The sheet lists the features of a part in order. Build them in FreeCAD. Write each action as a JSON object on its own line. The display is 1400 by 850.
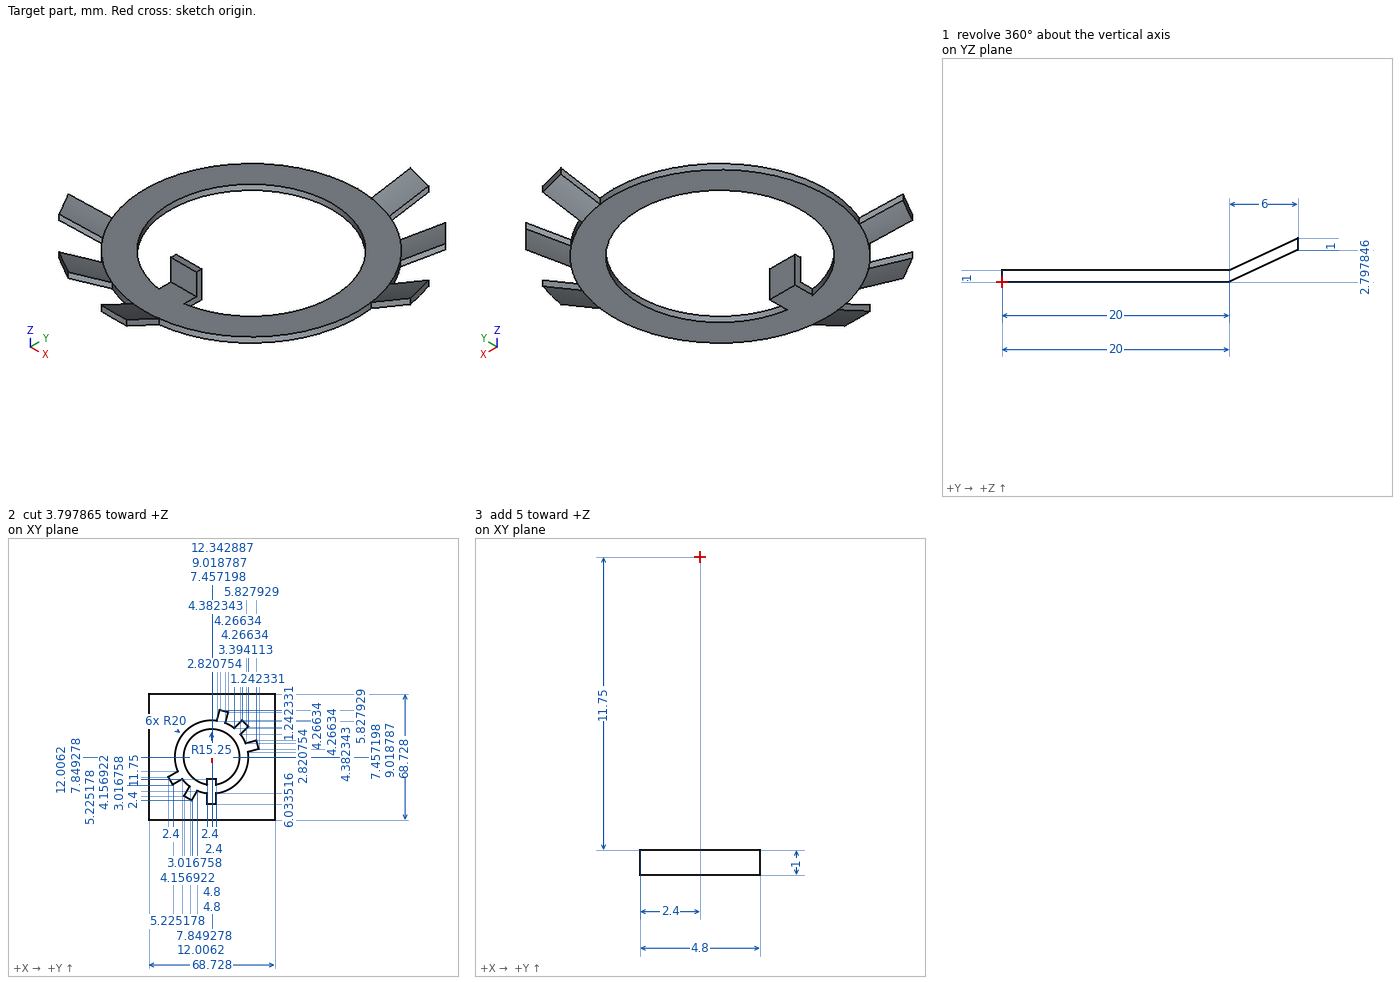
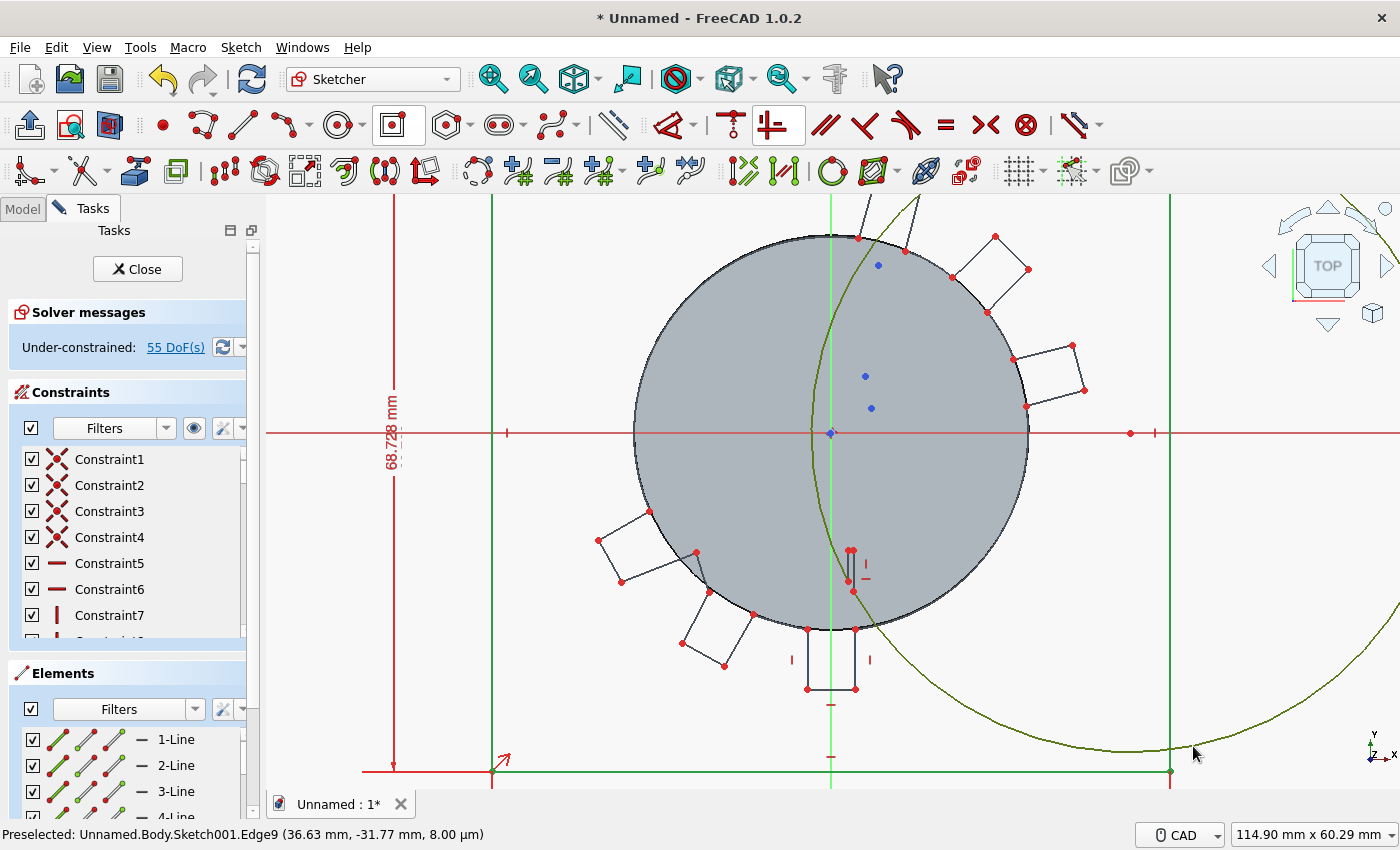
{"action": "left_click", "coordinate": [738, 260]}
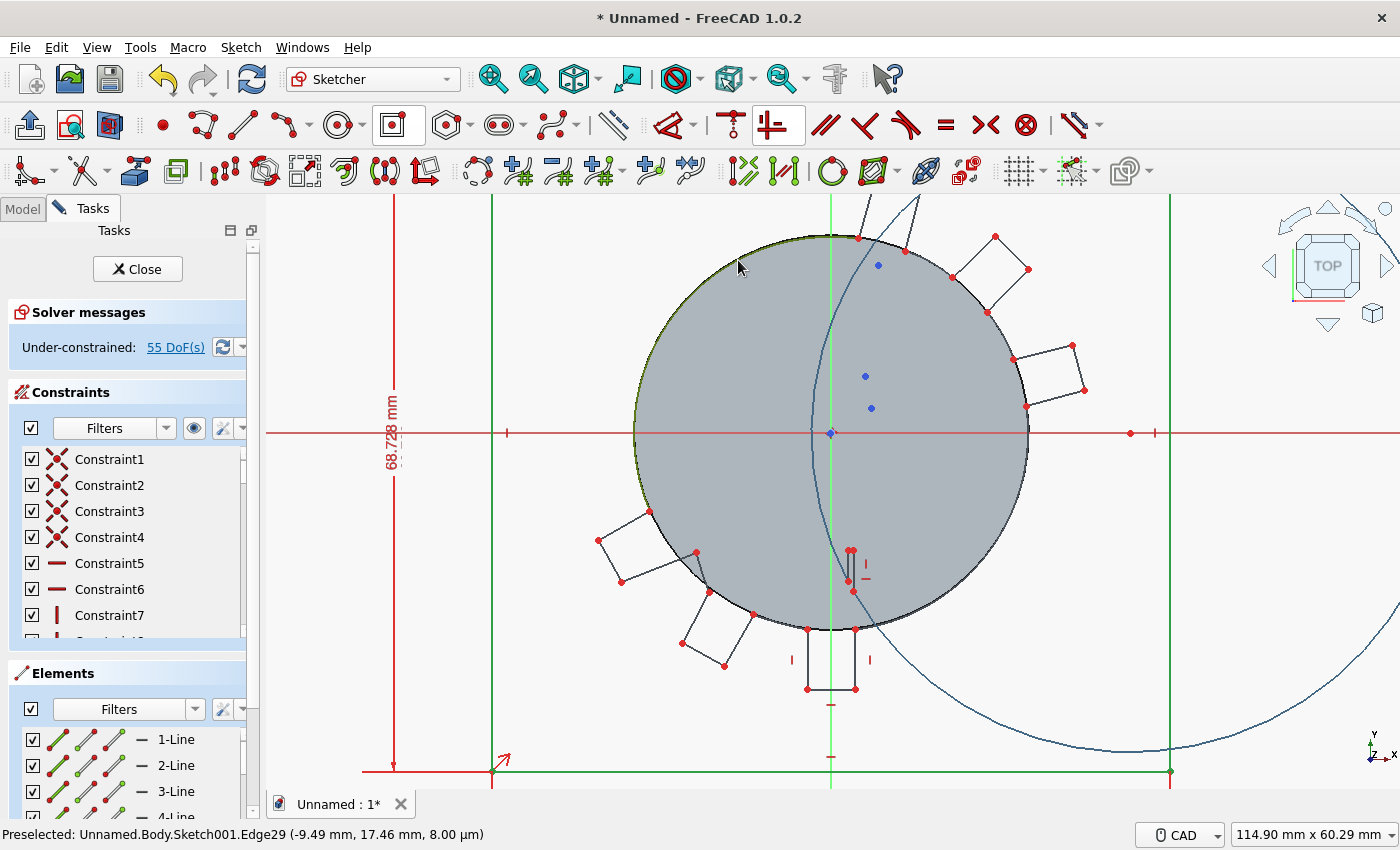
{"action": "left_click", "coordinate": [732, 126]}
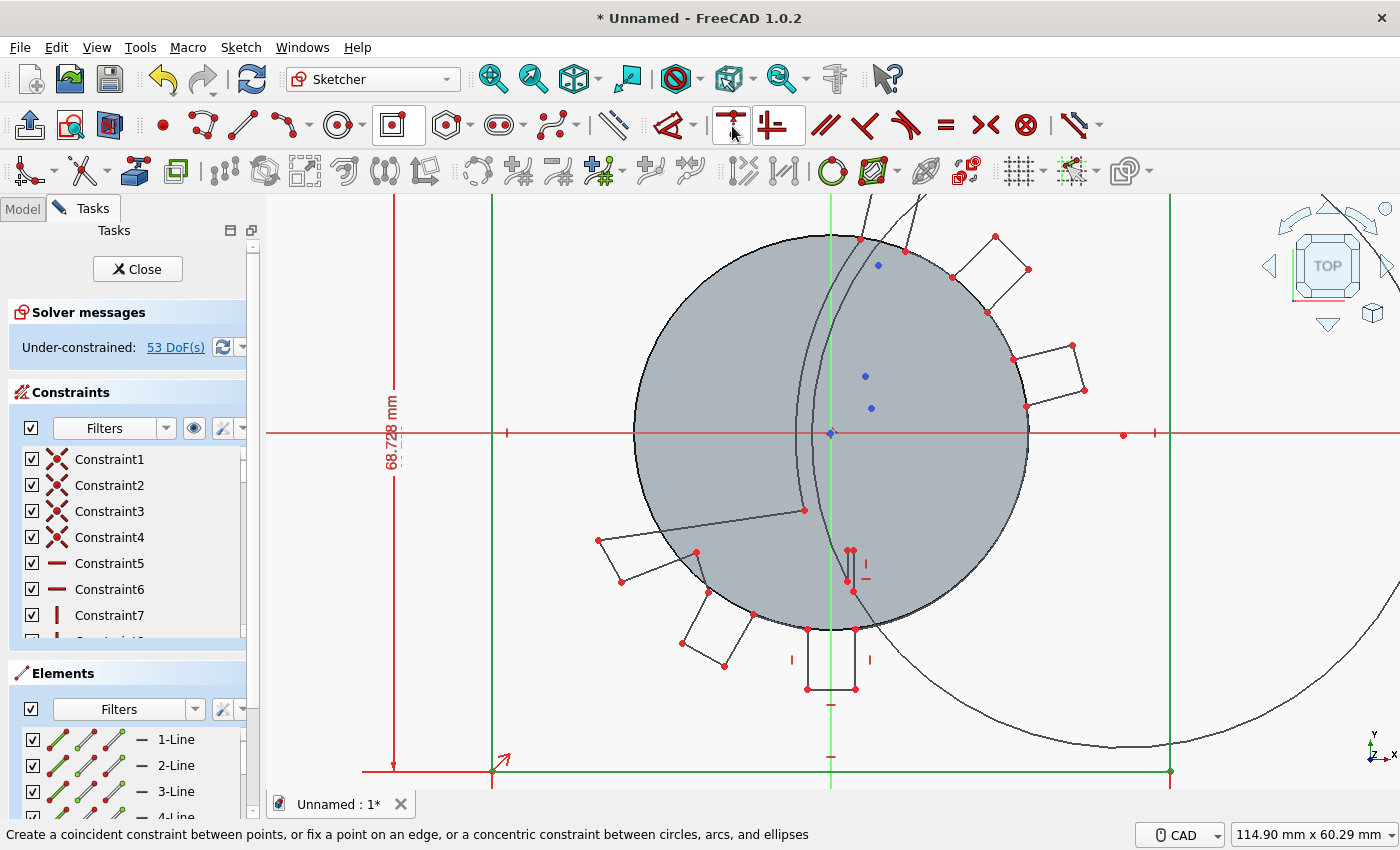
{"action": "left_click", "coordinate": [1186, 742]}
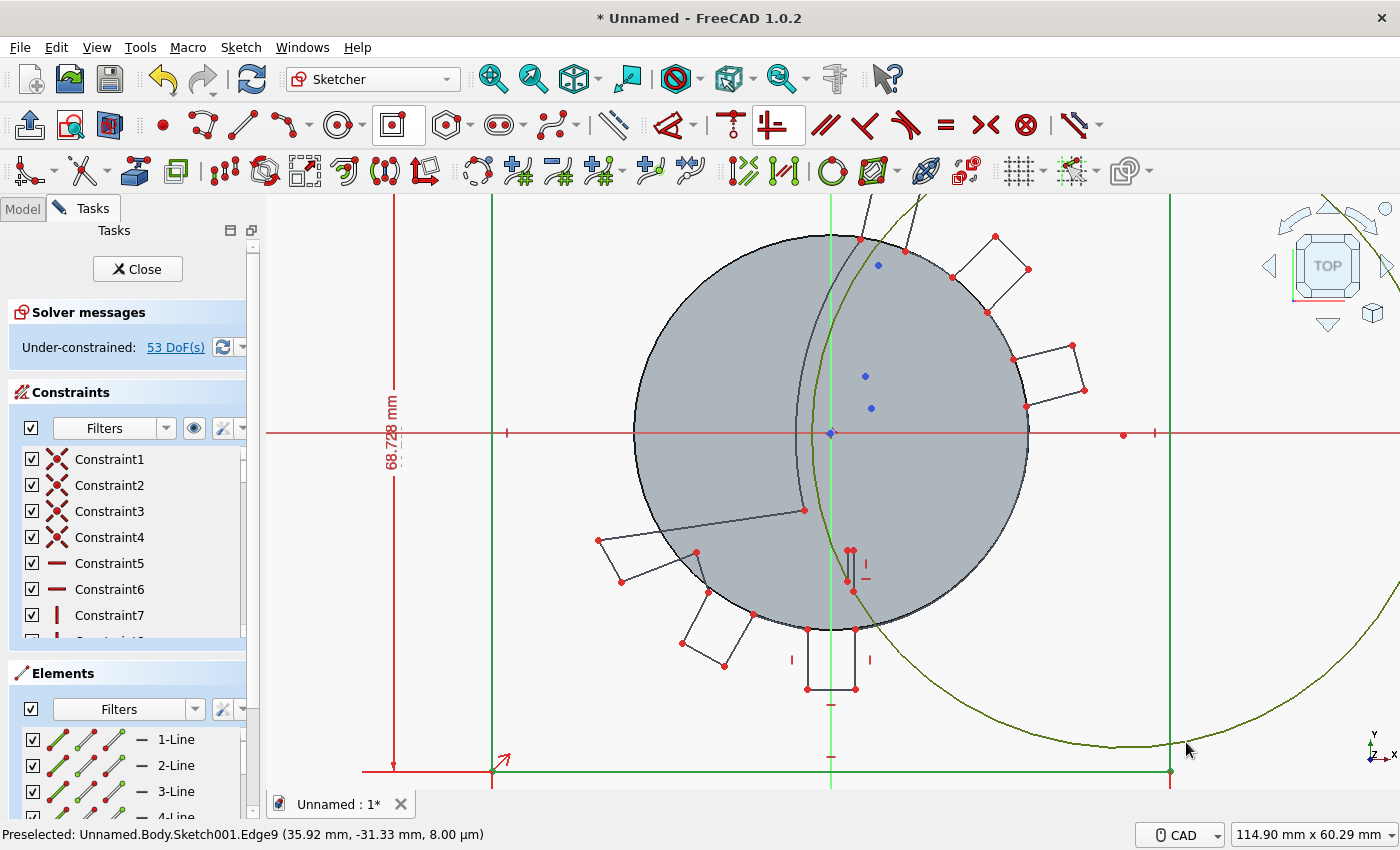
{"action": "left_click", "coordinate": [940, 268]}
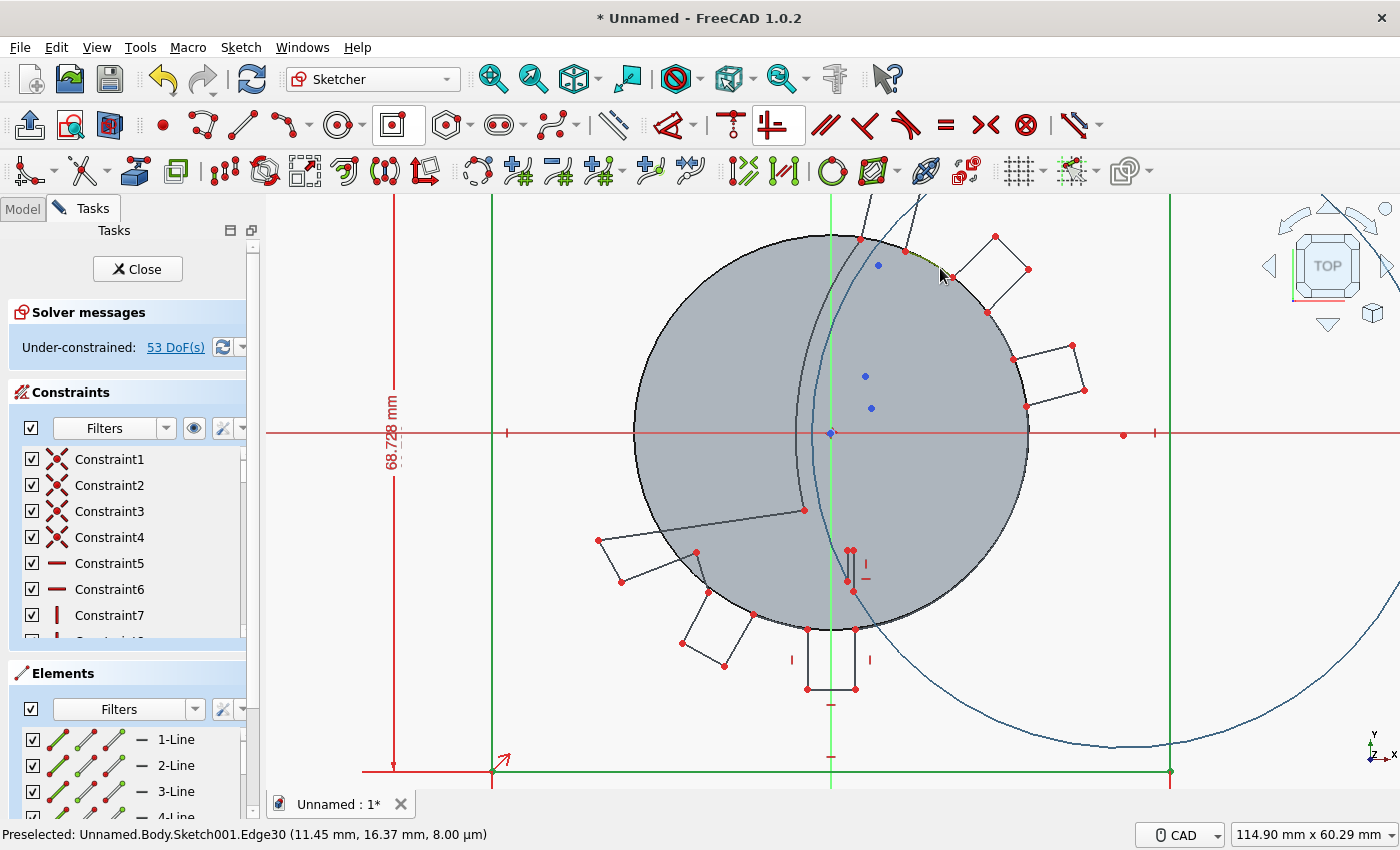
{"action": "left_click", "coordinate": [732, 126]}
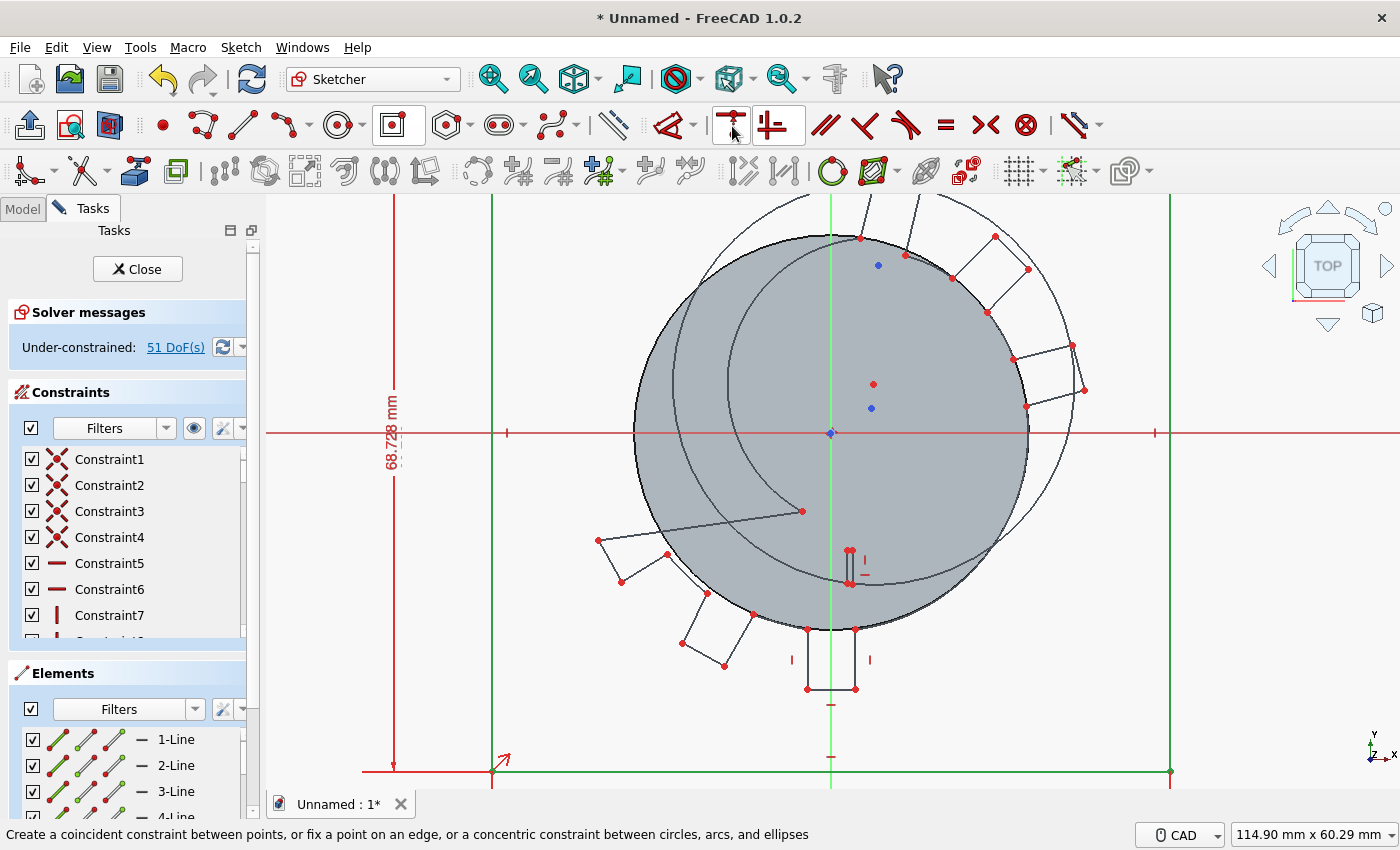
{"action": "left_click", "coordinate": [692, 299]}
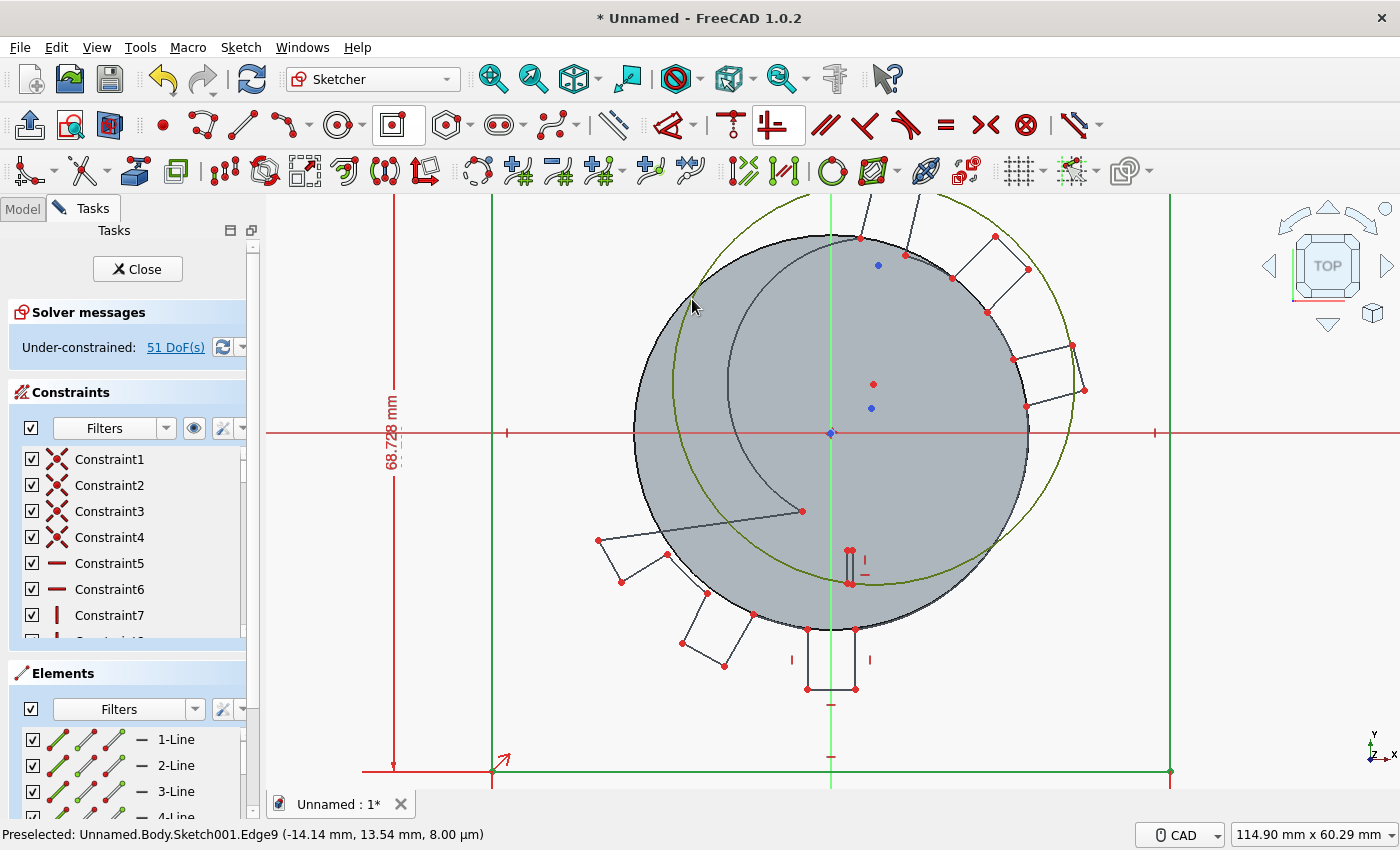
{"action": "left_click", "coordinate": [1008, 344]}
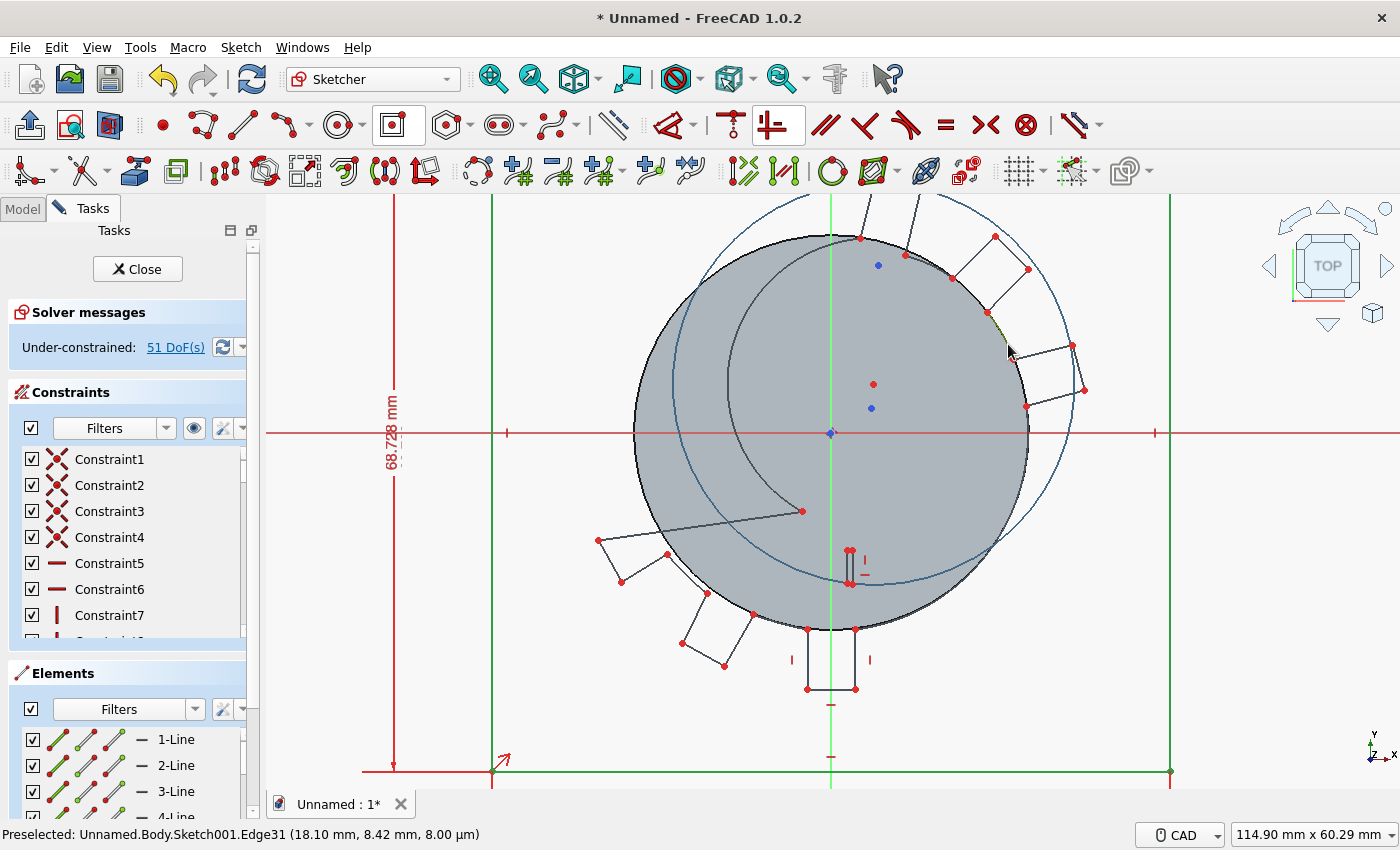
{"action": "left_click", "coordinate": [732, 126]}